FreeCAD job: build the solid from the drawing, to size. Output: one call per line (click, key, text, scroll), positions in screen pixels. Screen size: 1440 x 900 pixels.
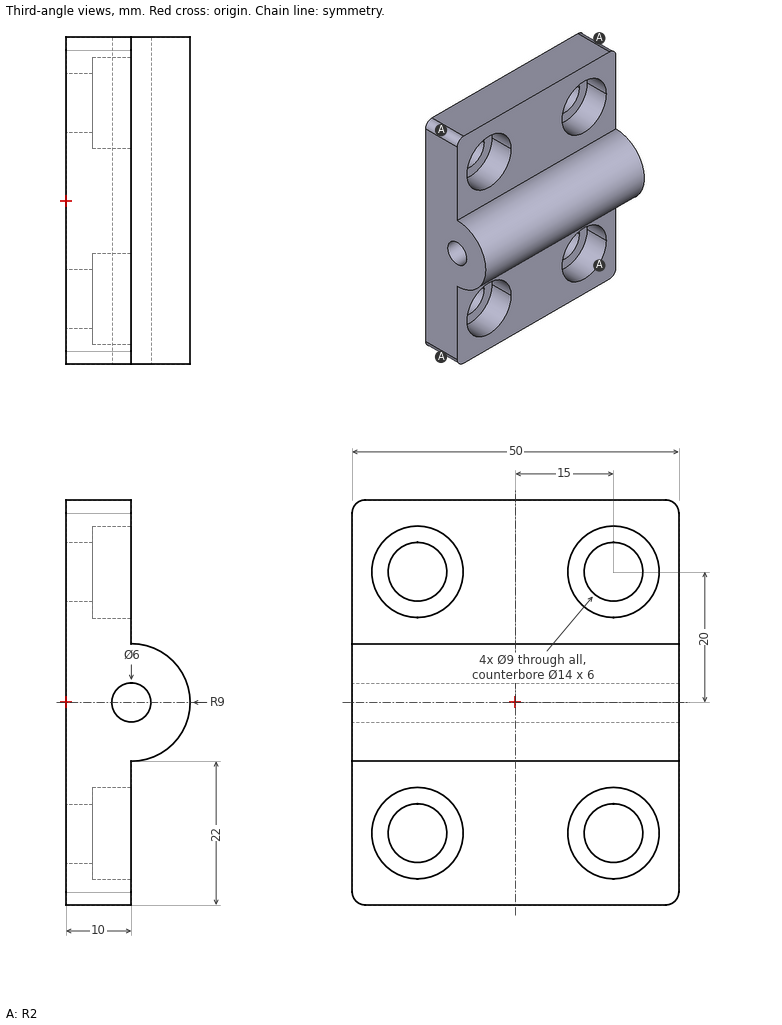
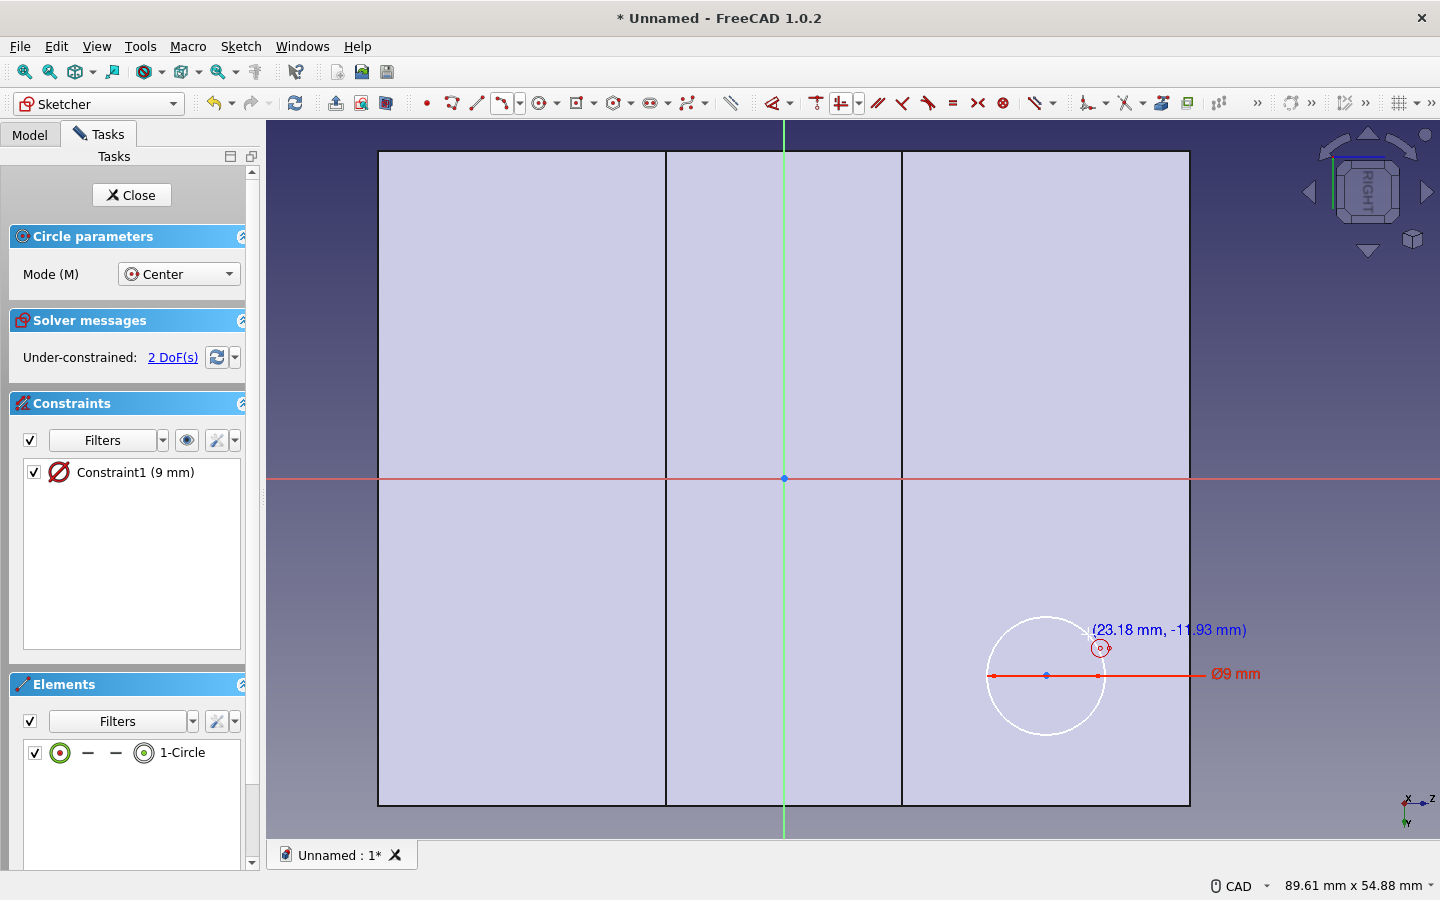
click(1046, 282)
move(1088, 240)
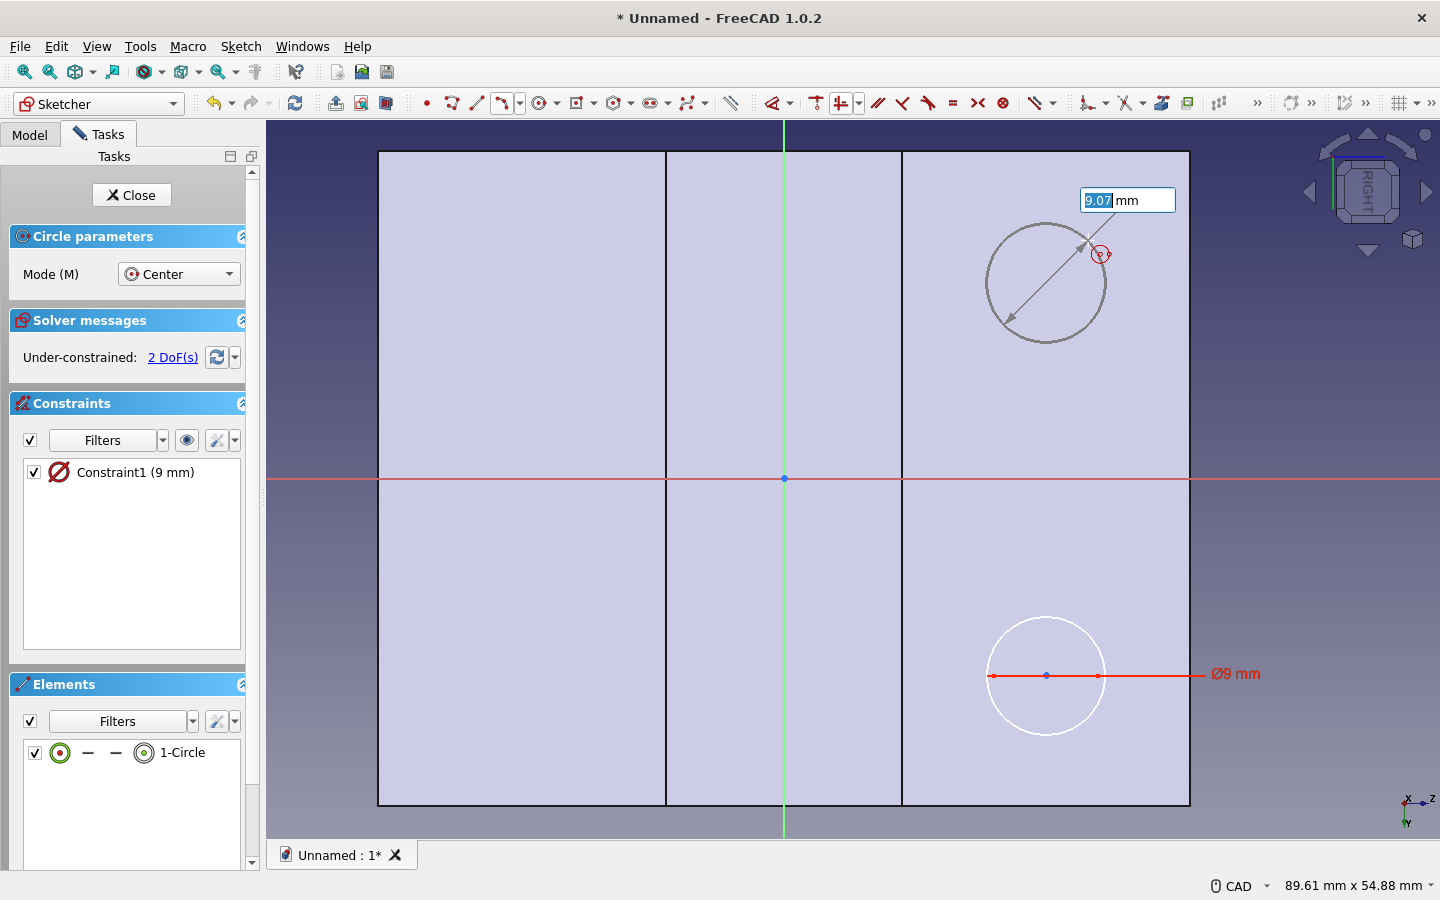
text(9)
key(Return)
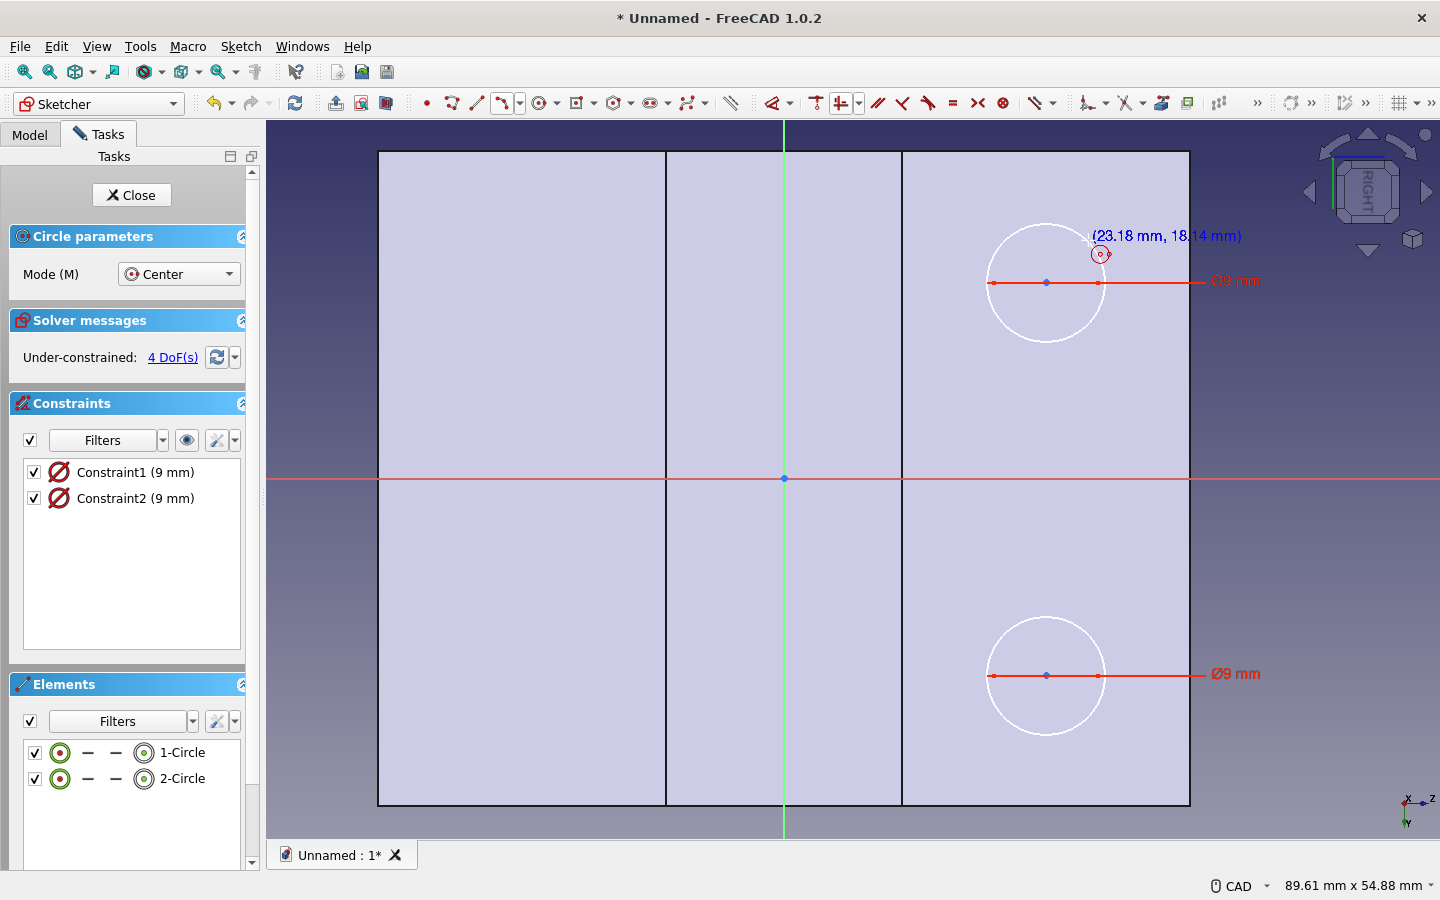
click(522, 282)
move(564, 240)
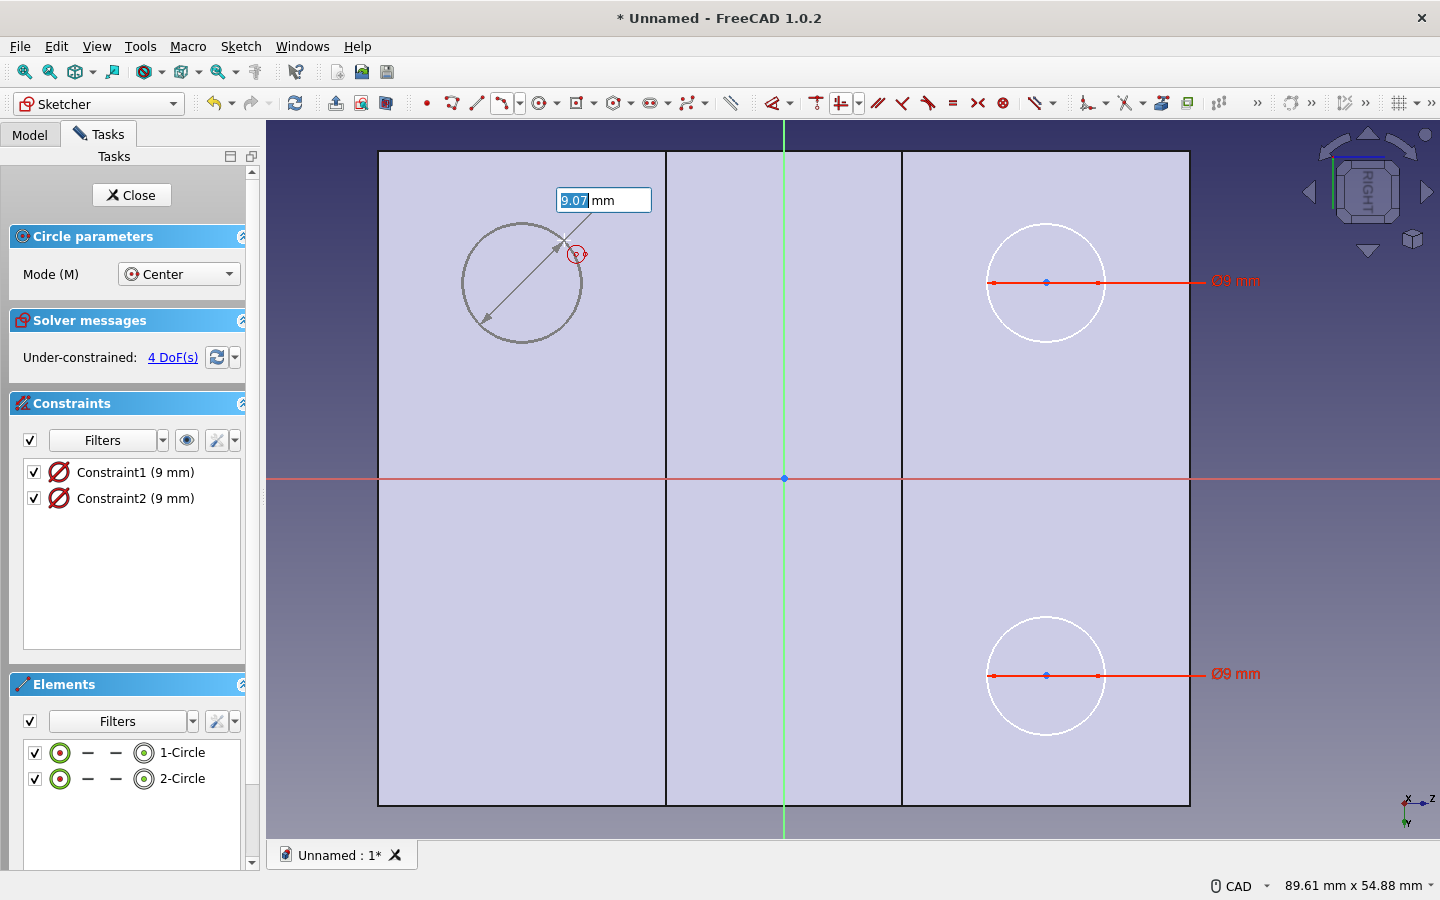
text(9)
key(Return)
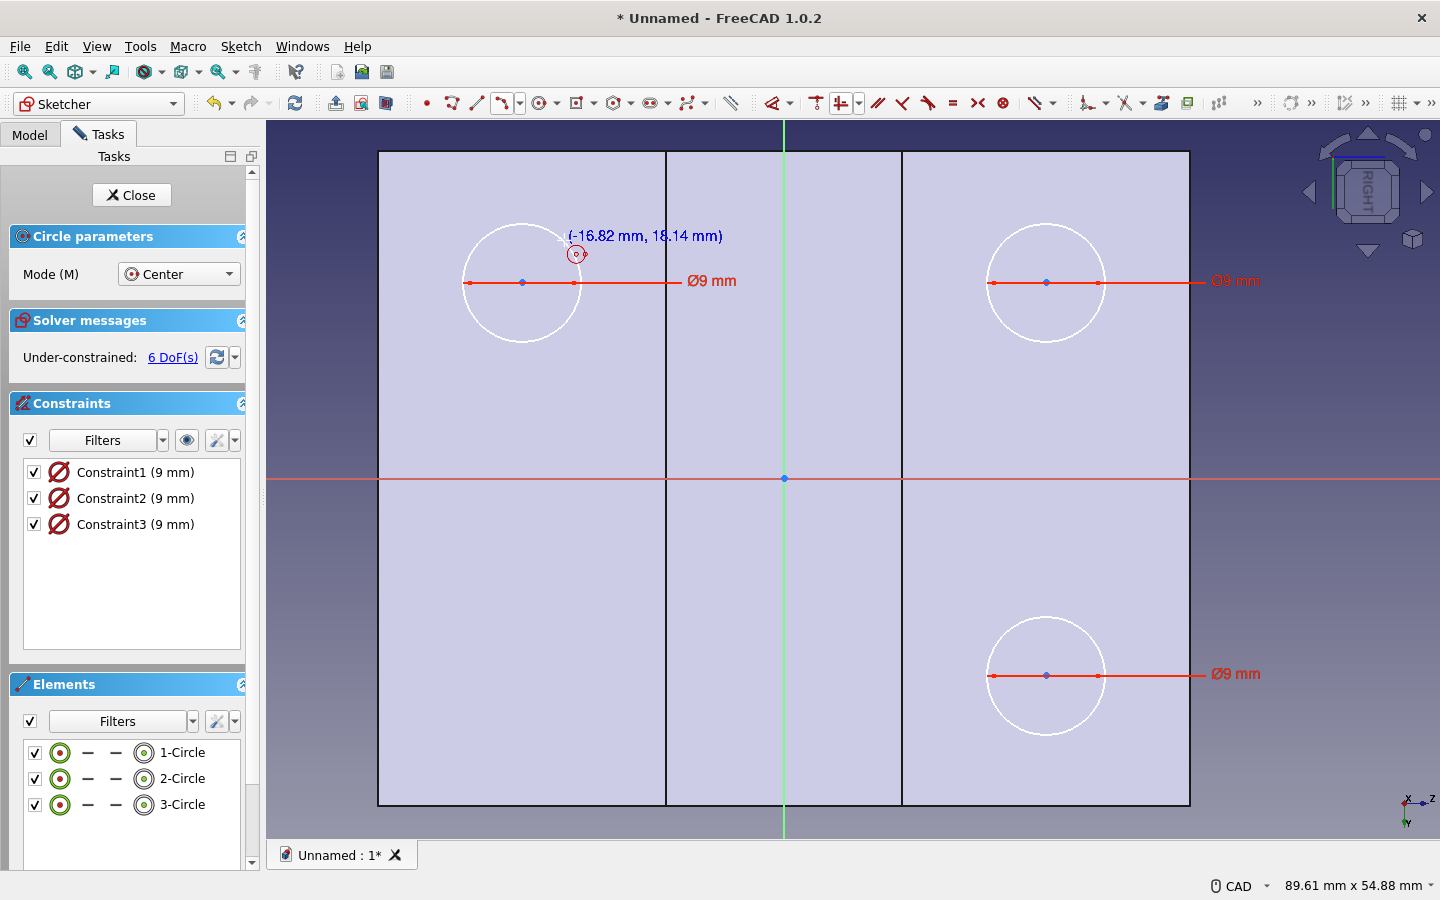
click(522, 675)
move(564, 634)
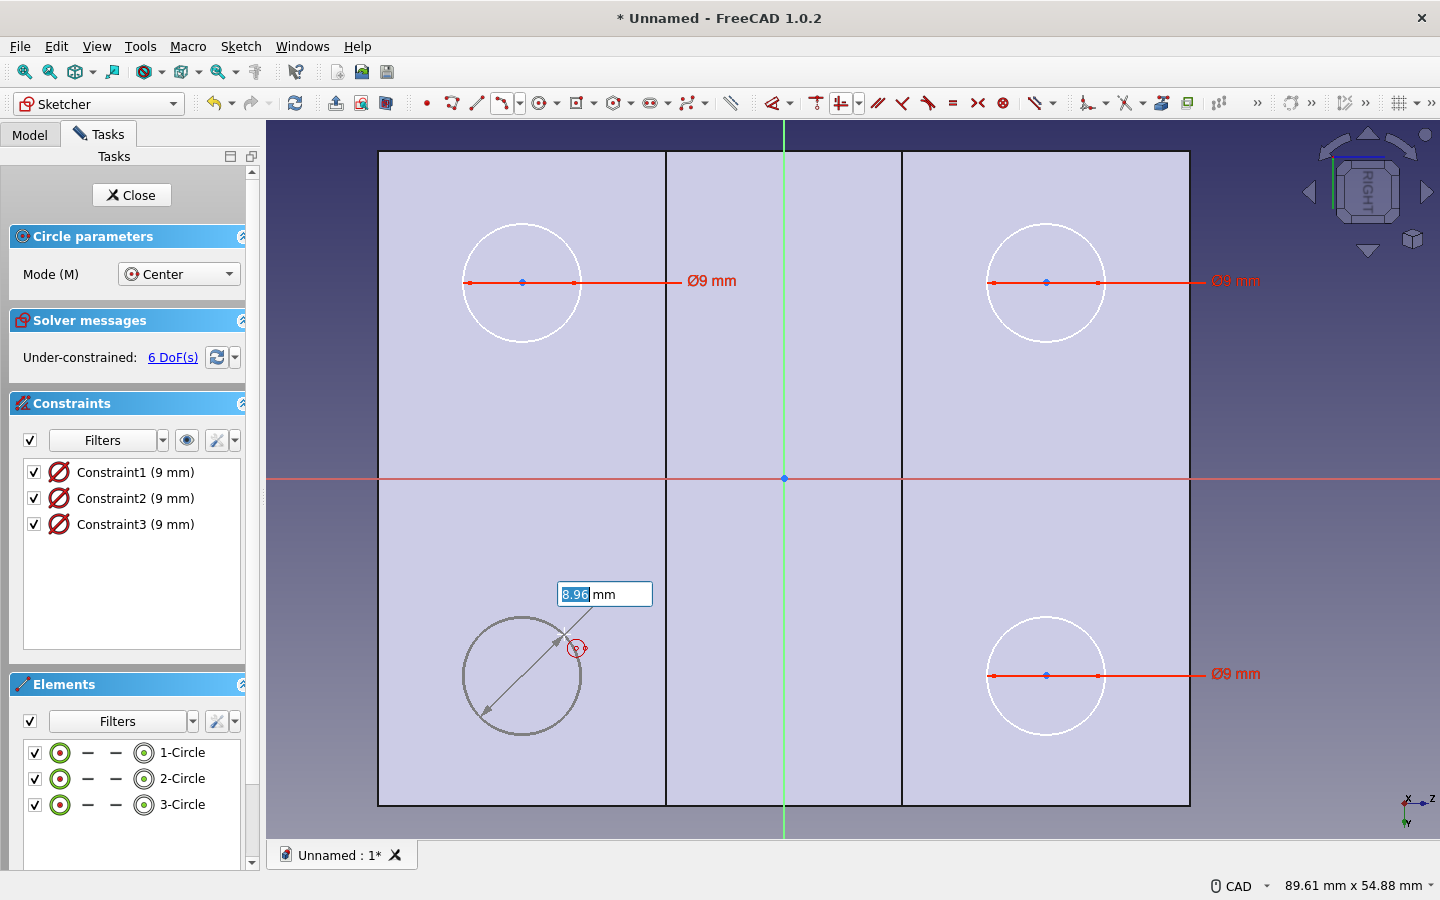
text(9)
key(Return)
key(Escape)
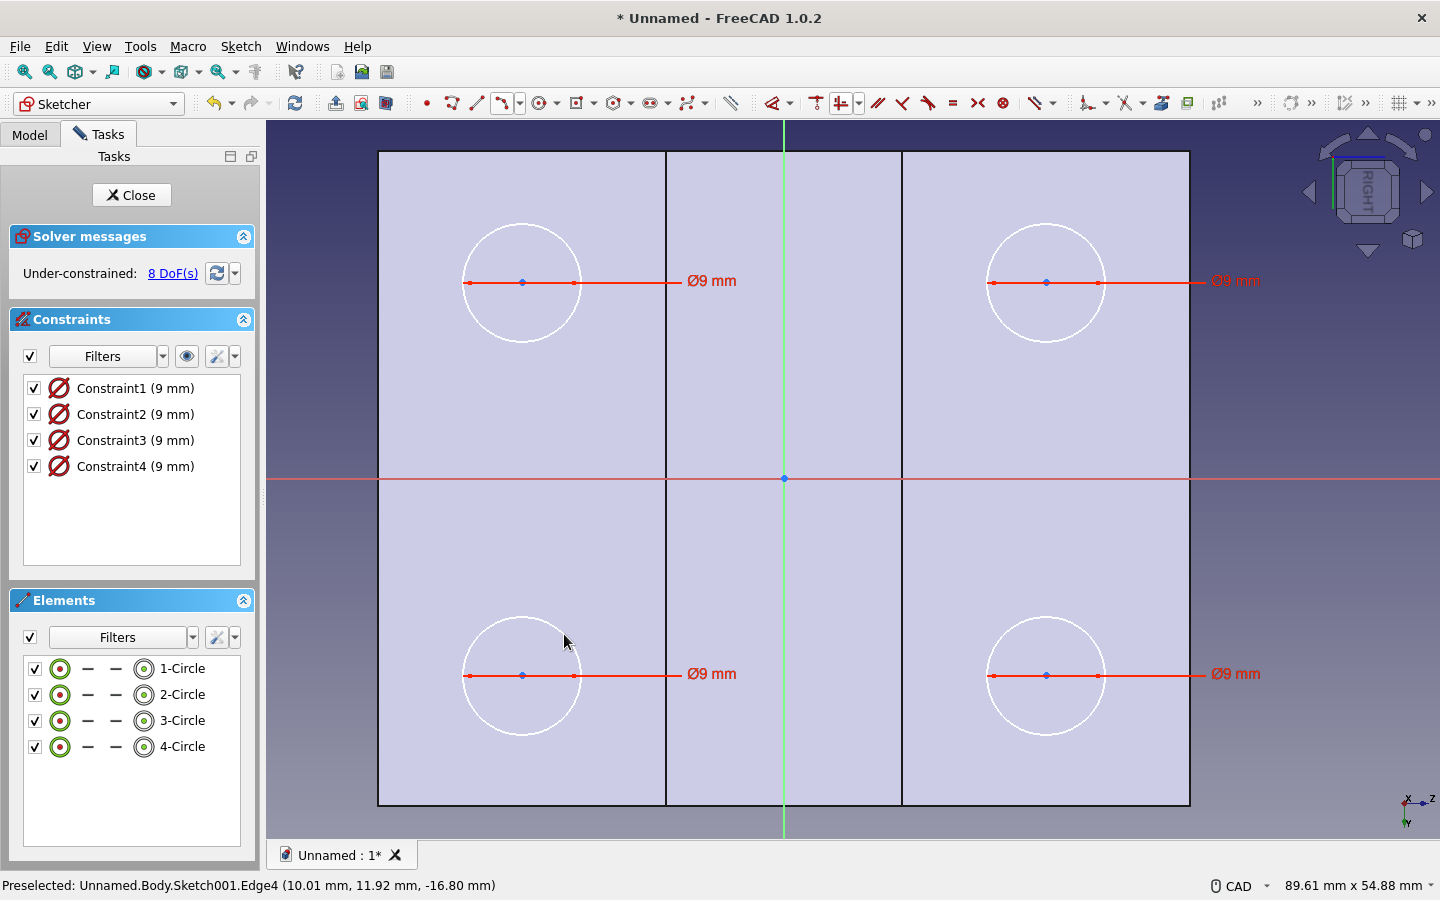
click(1046, 676)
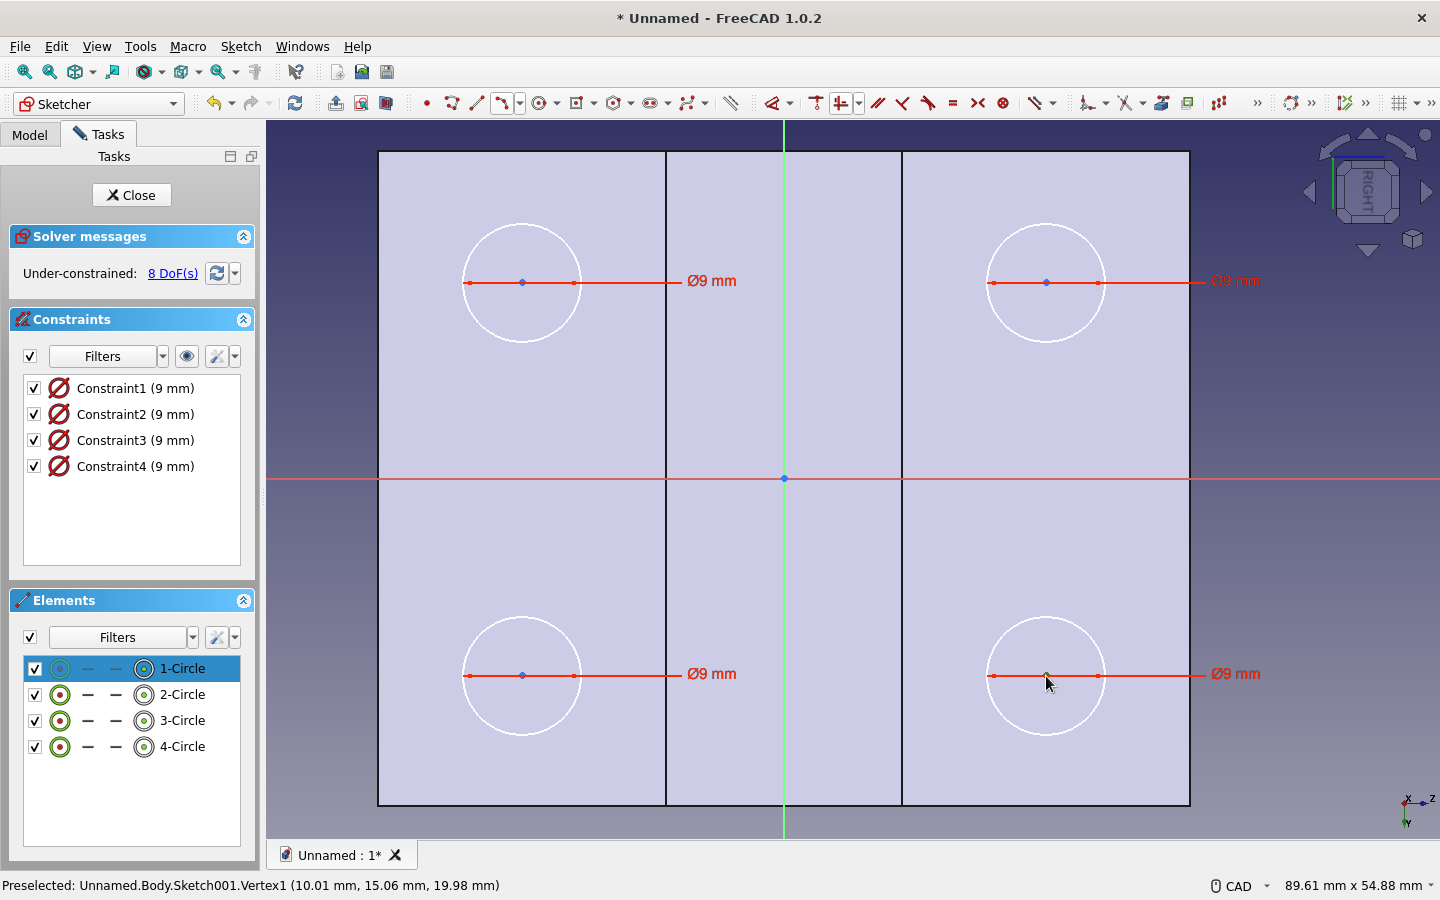
click(1046, 283)